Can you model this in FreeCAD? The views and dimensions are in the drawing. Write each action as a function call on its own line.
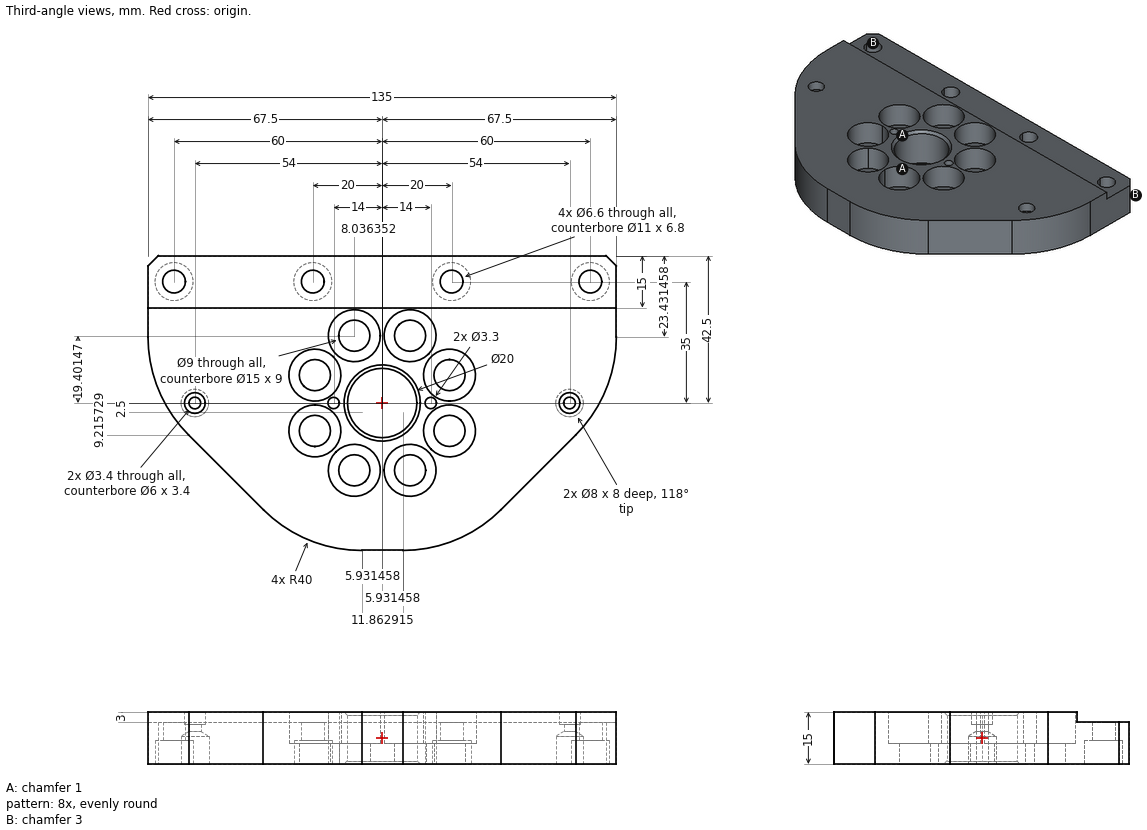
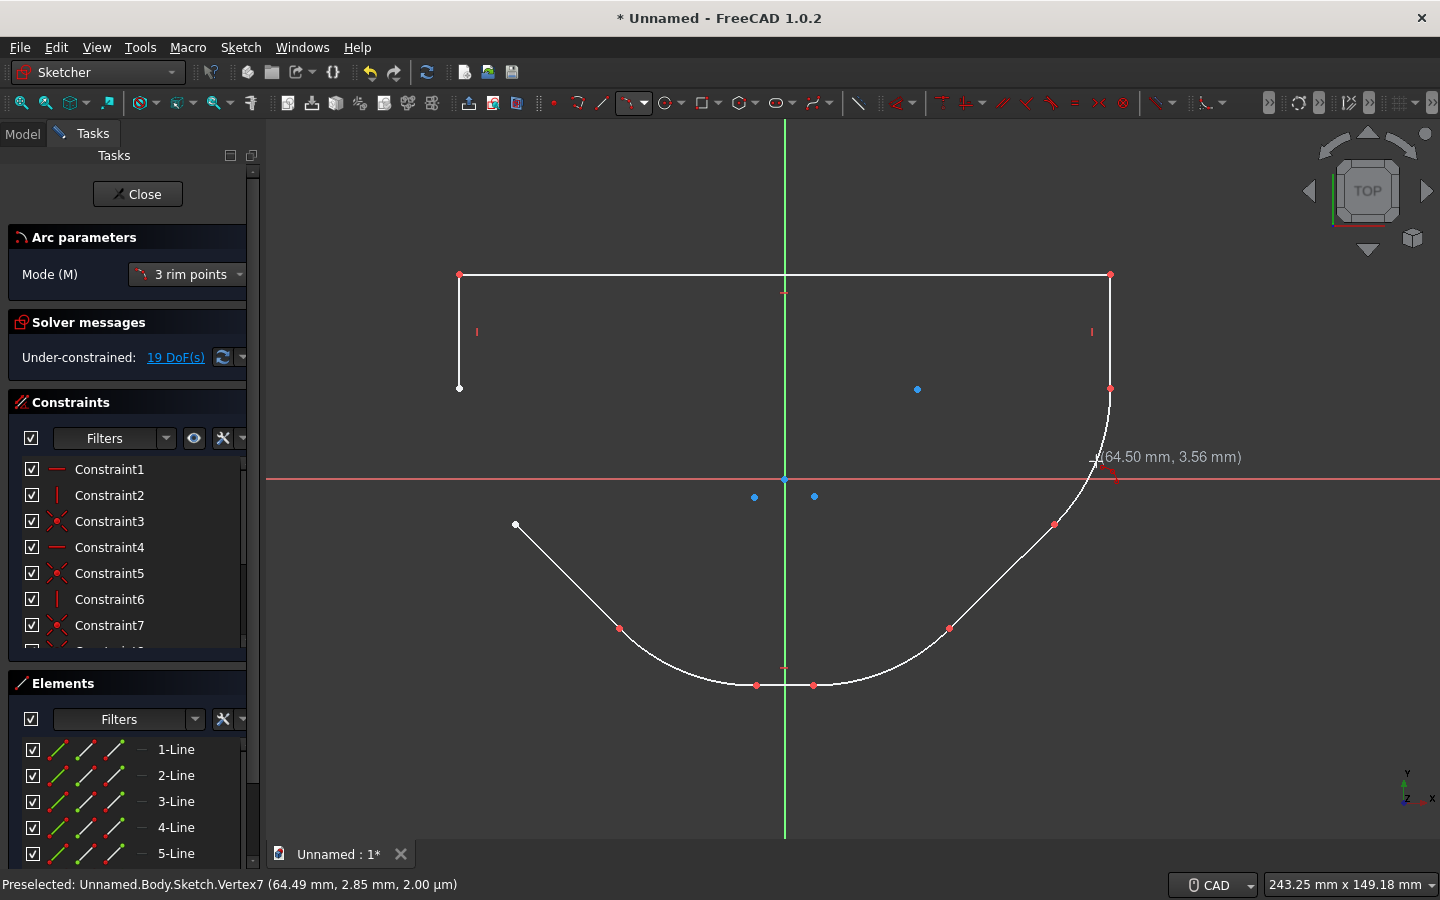
click(459, 388)
click(516, 525)
click(474, 461)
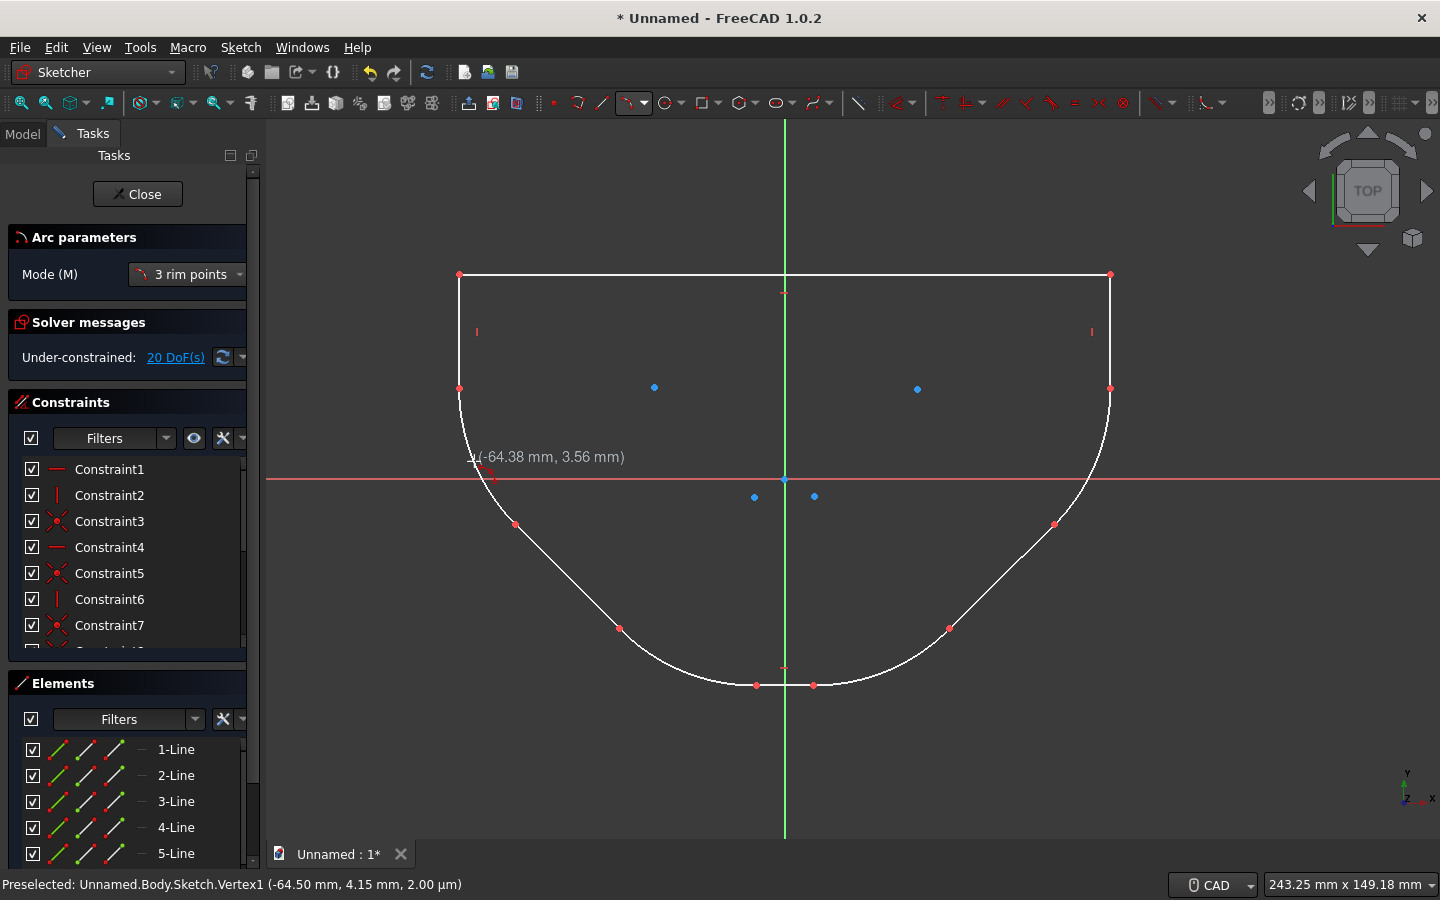
click(666, 104)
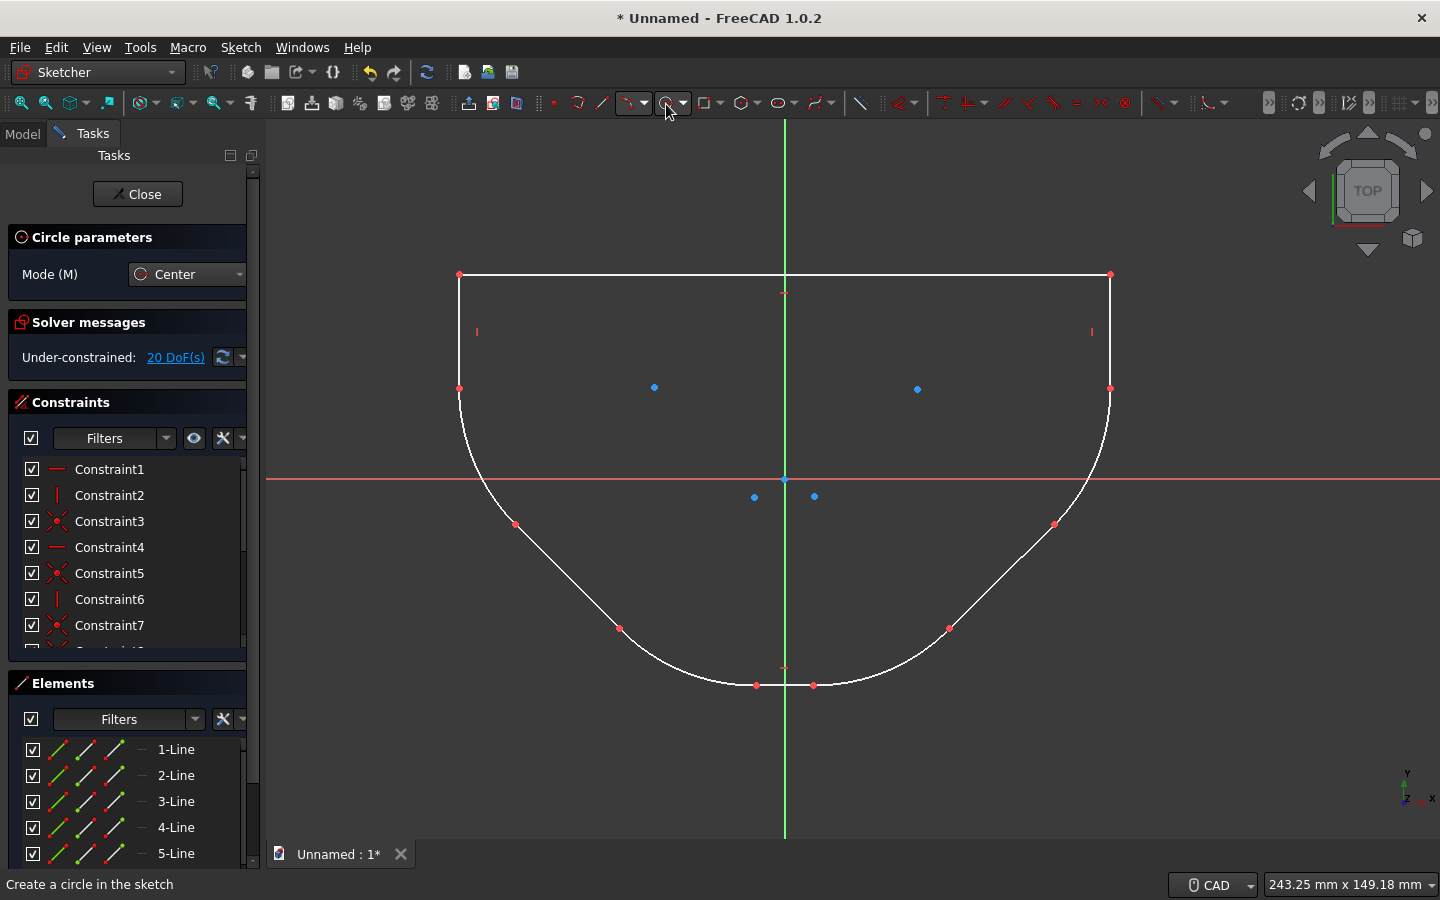
click(785, 479)
move(819, 445)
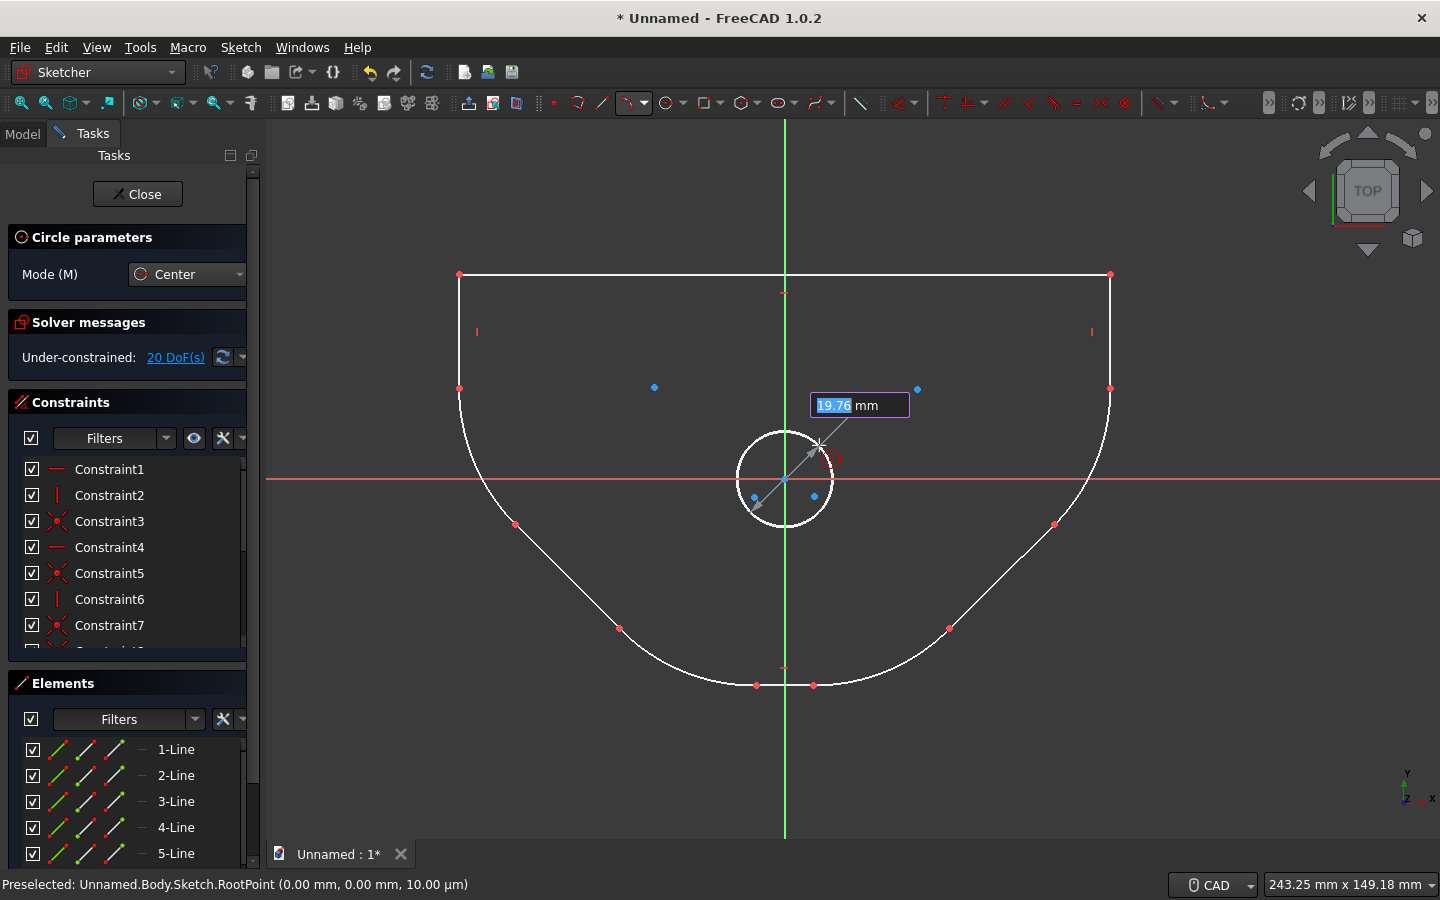
text(20)
key(Return)
key(Escape)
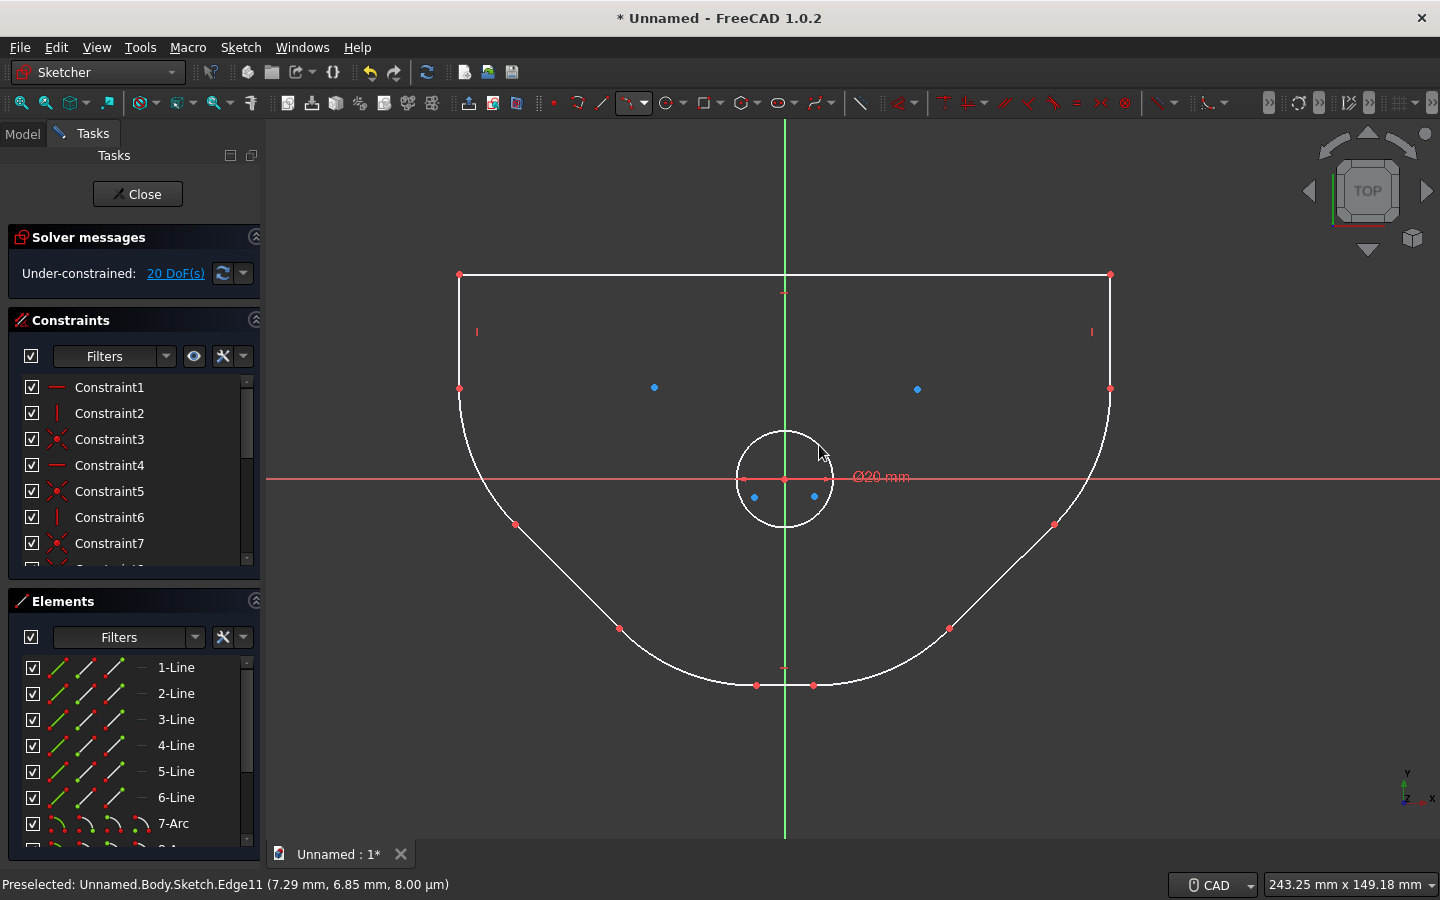
click(547, 556)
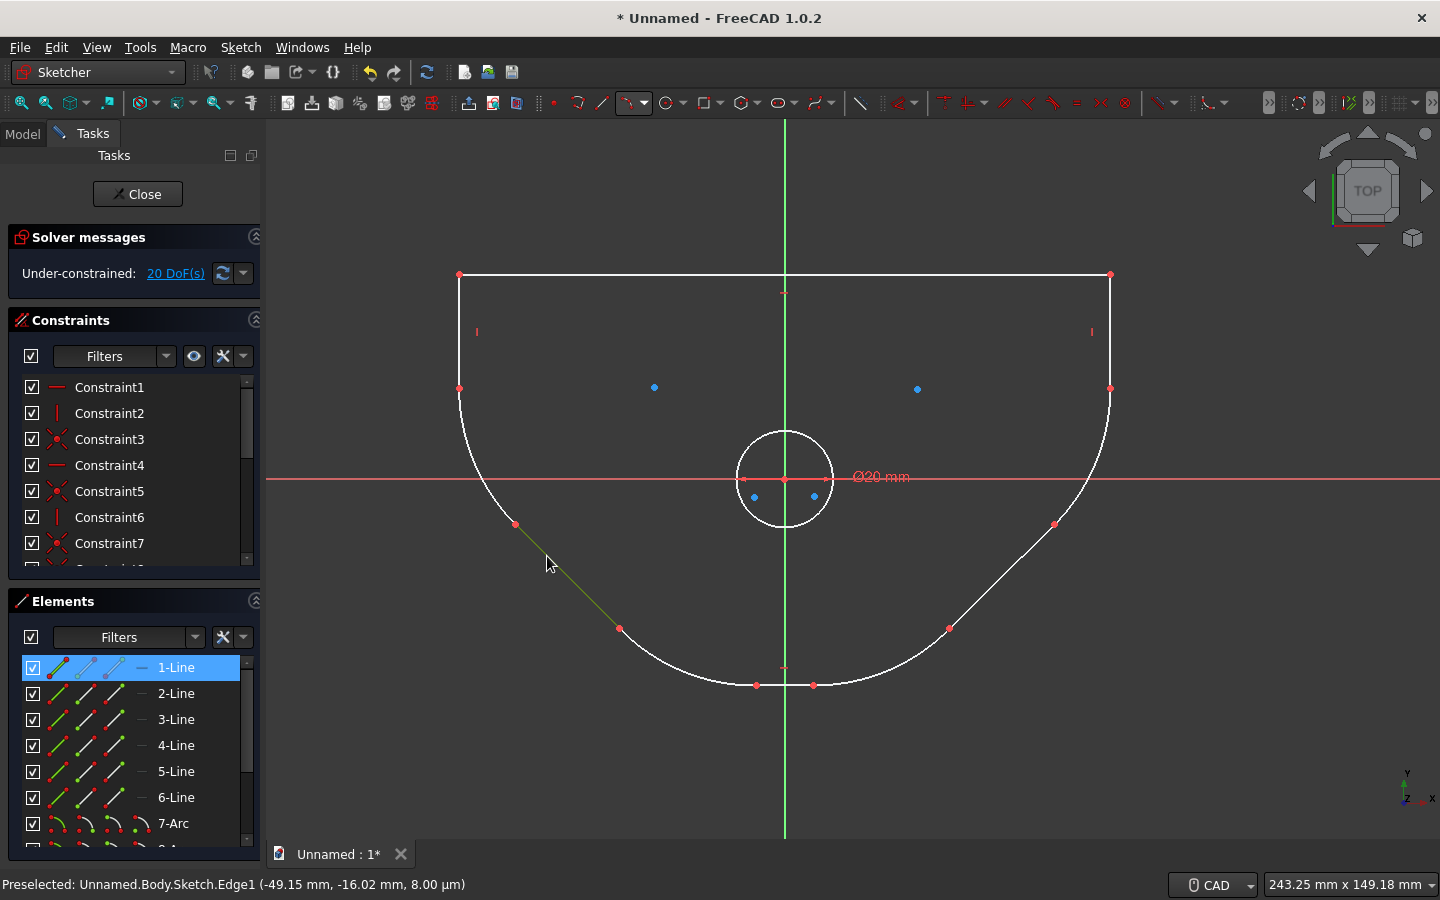
click(655, 657)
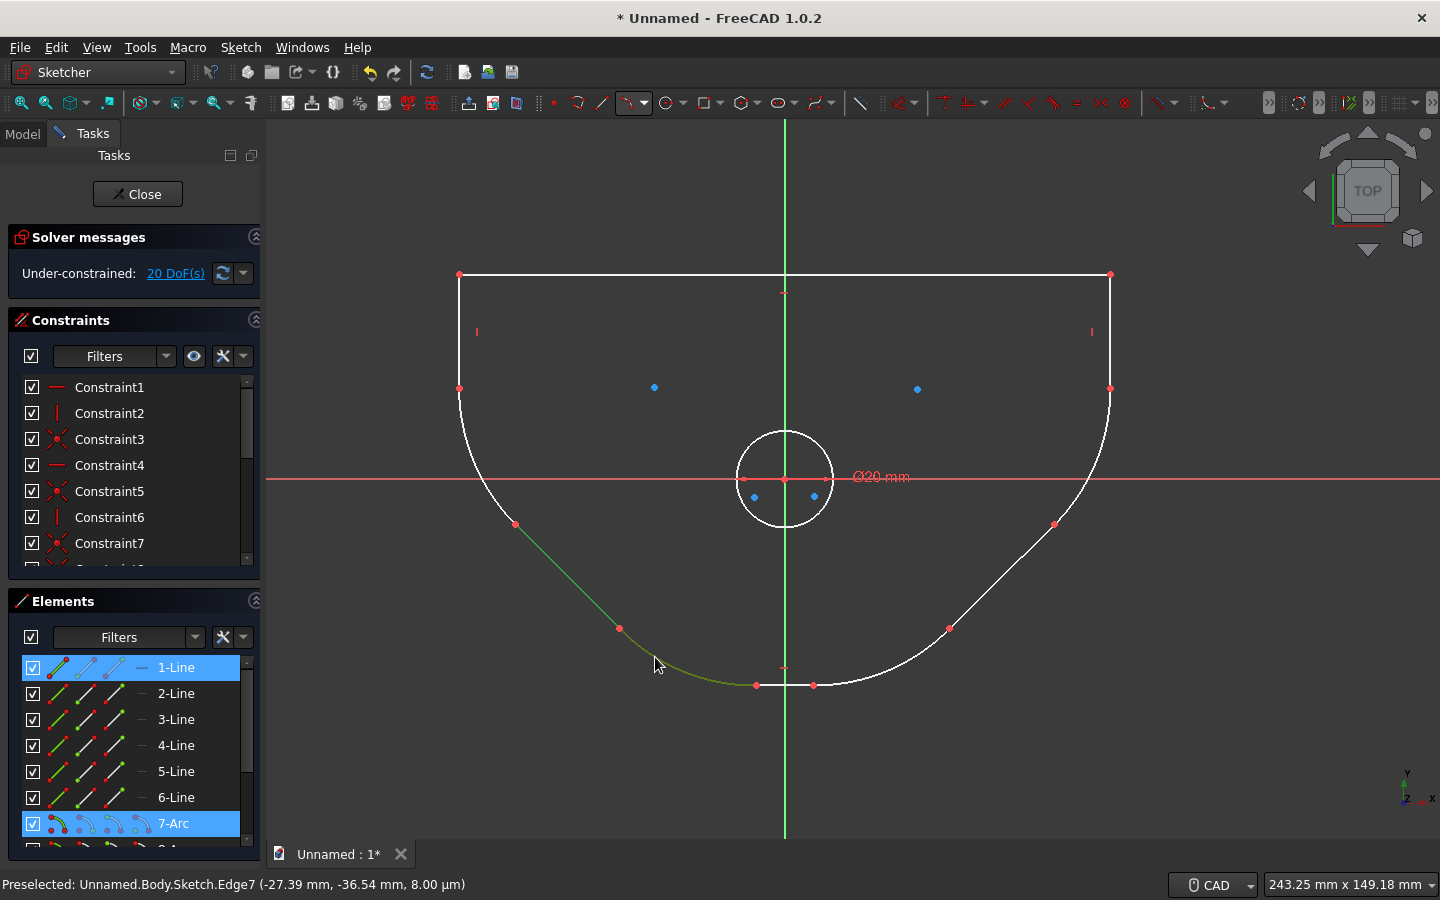
click(1054, 104)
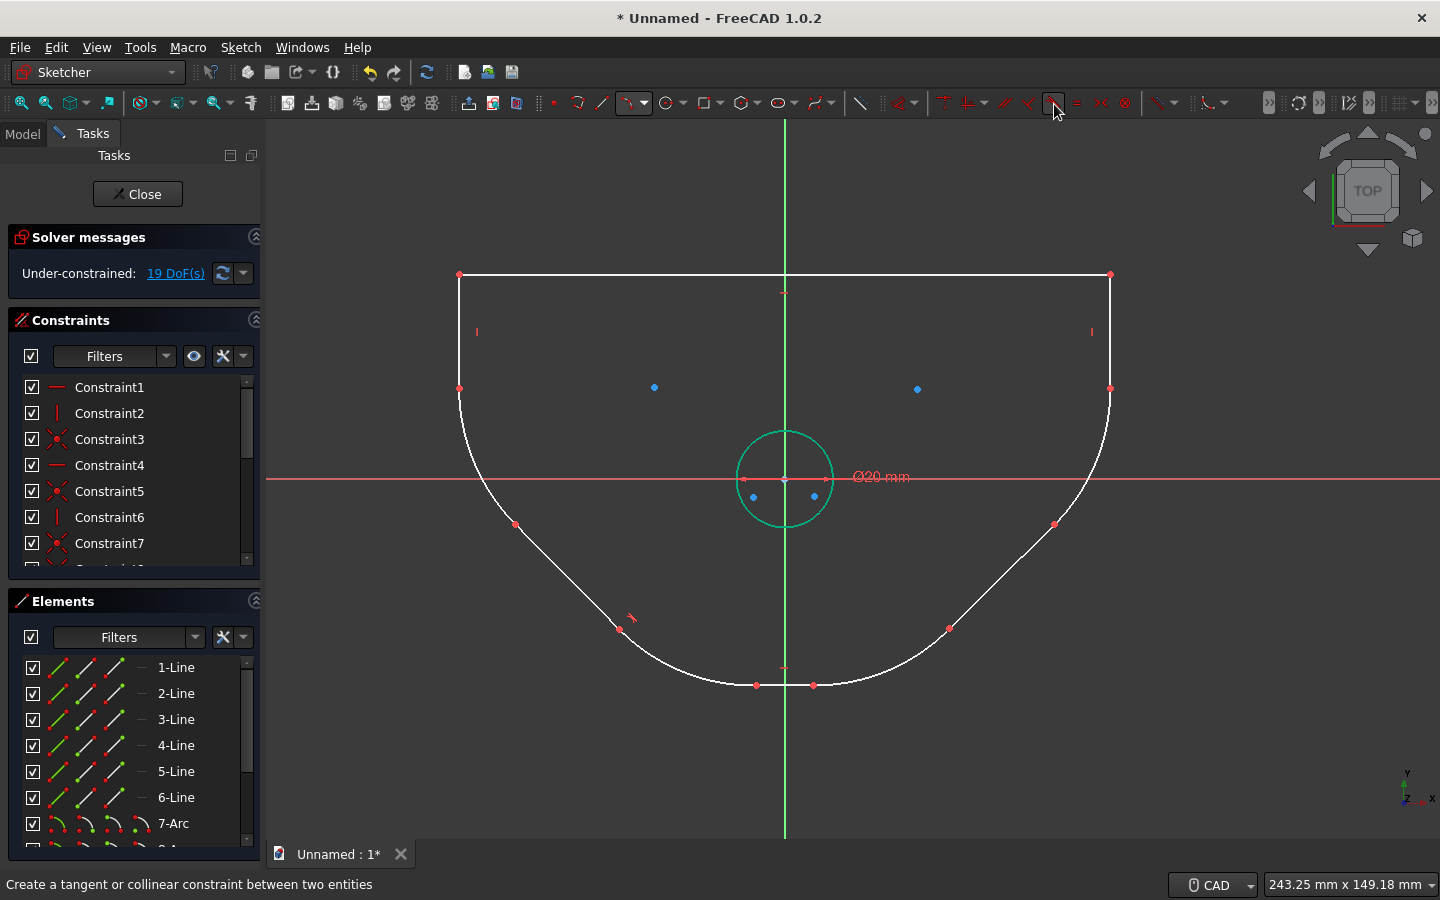
click(547, 556)